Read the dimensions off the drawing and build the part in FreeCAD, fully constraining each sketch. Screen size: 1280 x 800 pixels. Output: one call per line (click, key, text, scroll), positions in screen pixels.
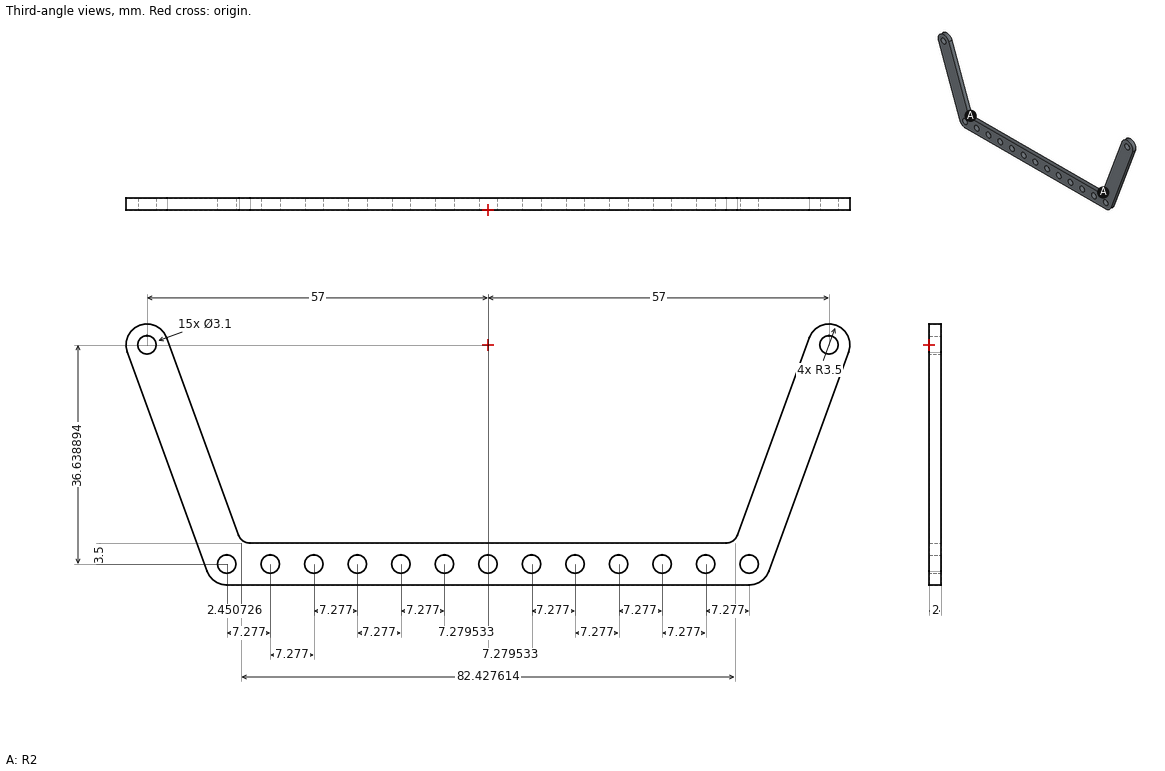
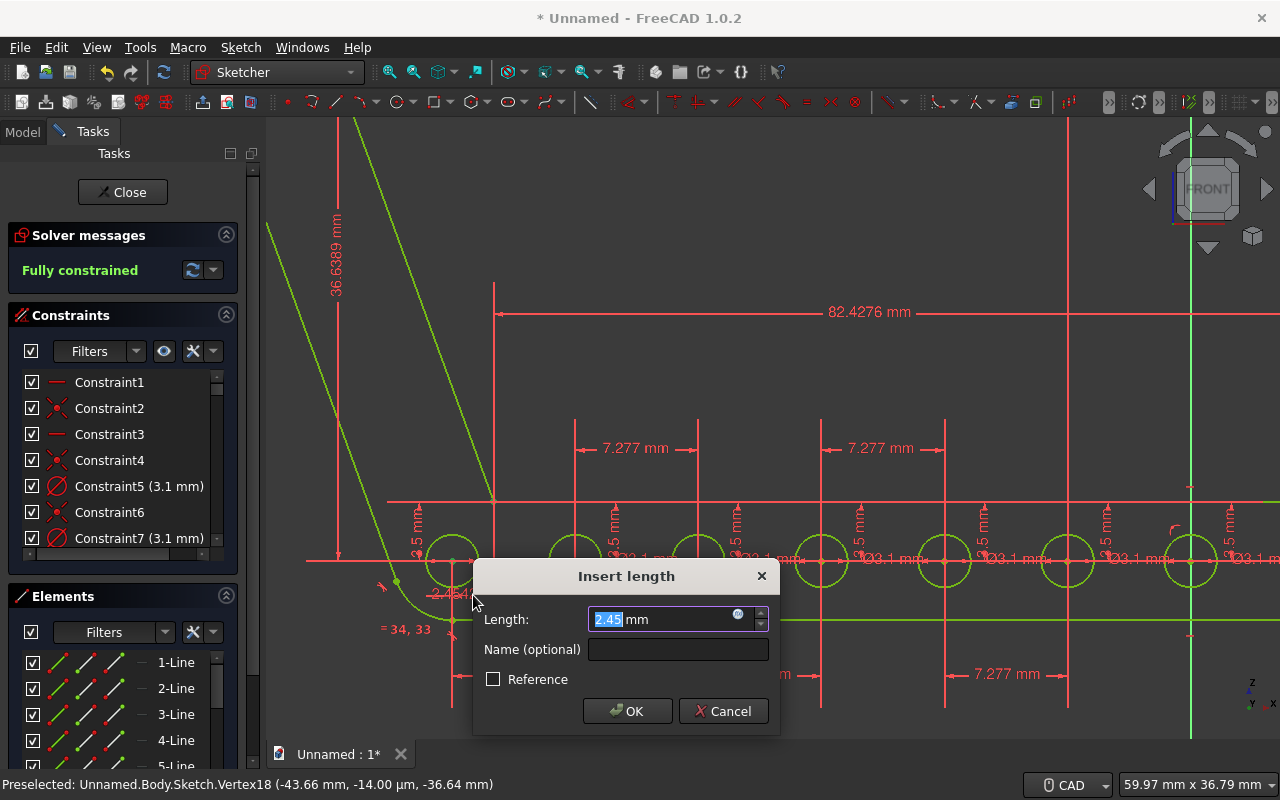
text(2.450726)
key(Return)
key(Escape)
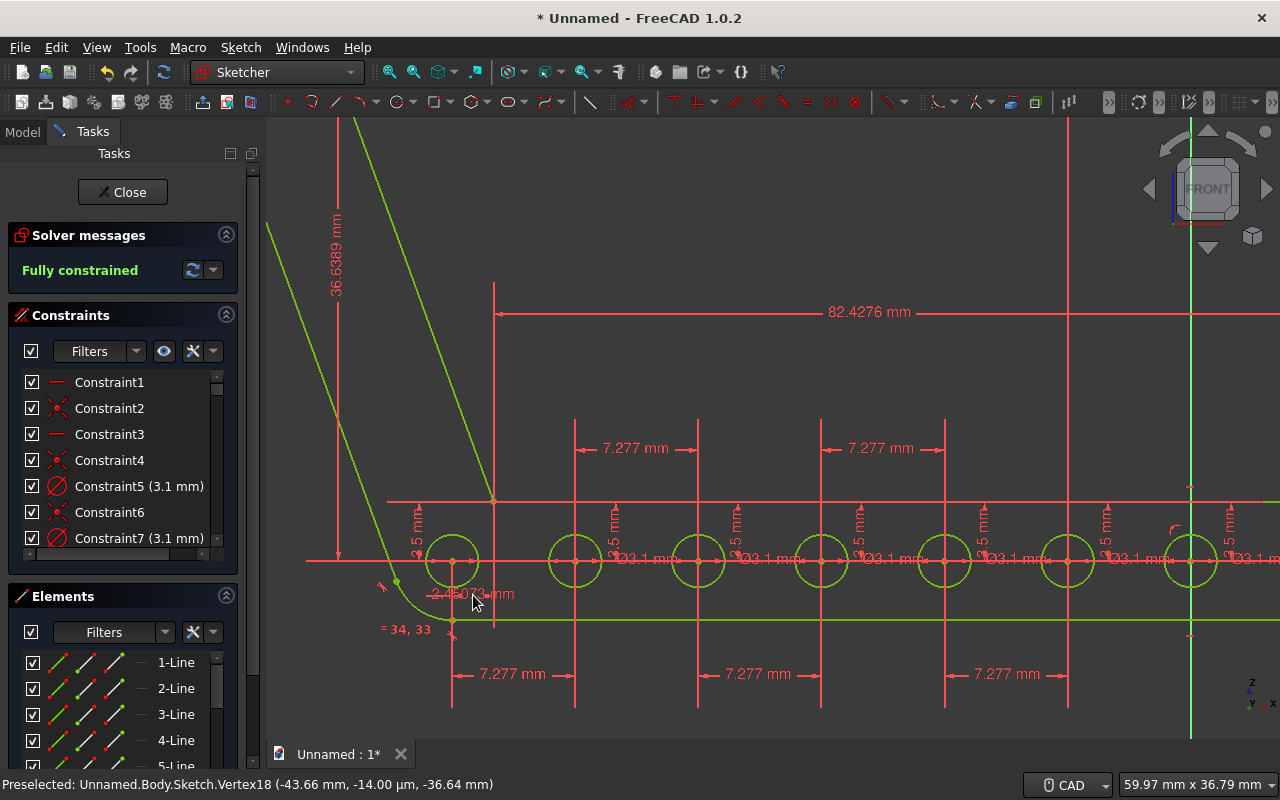
click(123, 192)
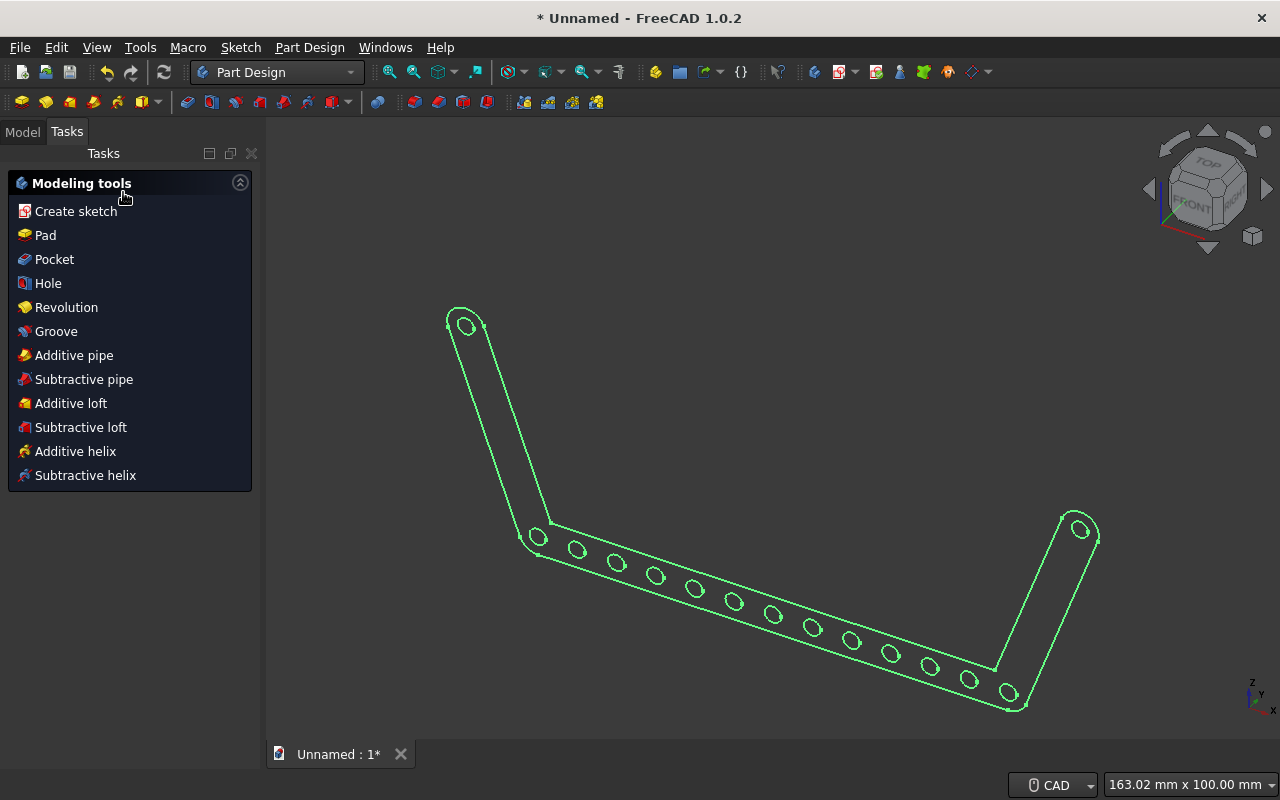
click(22, 102)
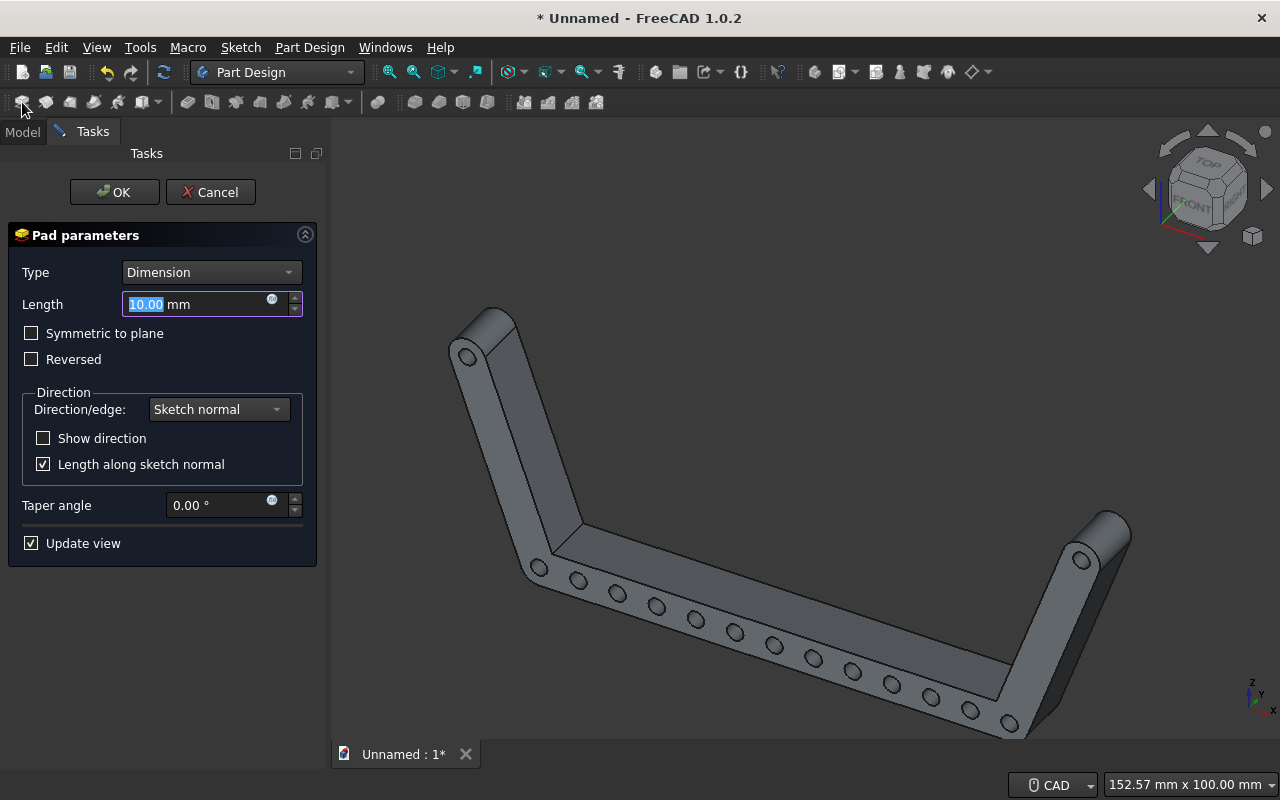
text(2)
key(Tab)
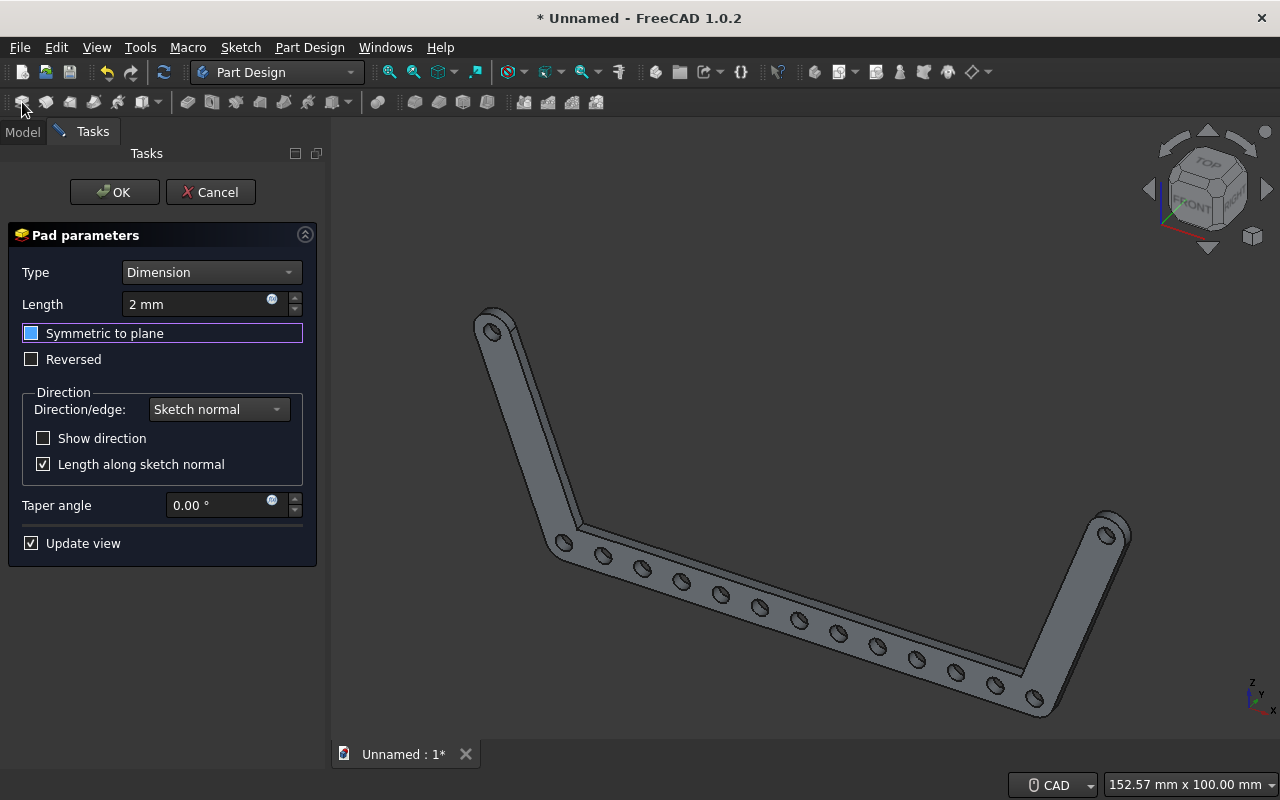
click(30, 359)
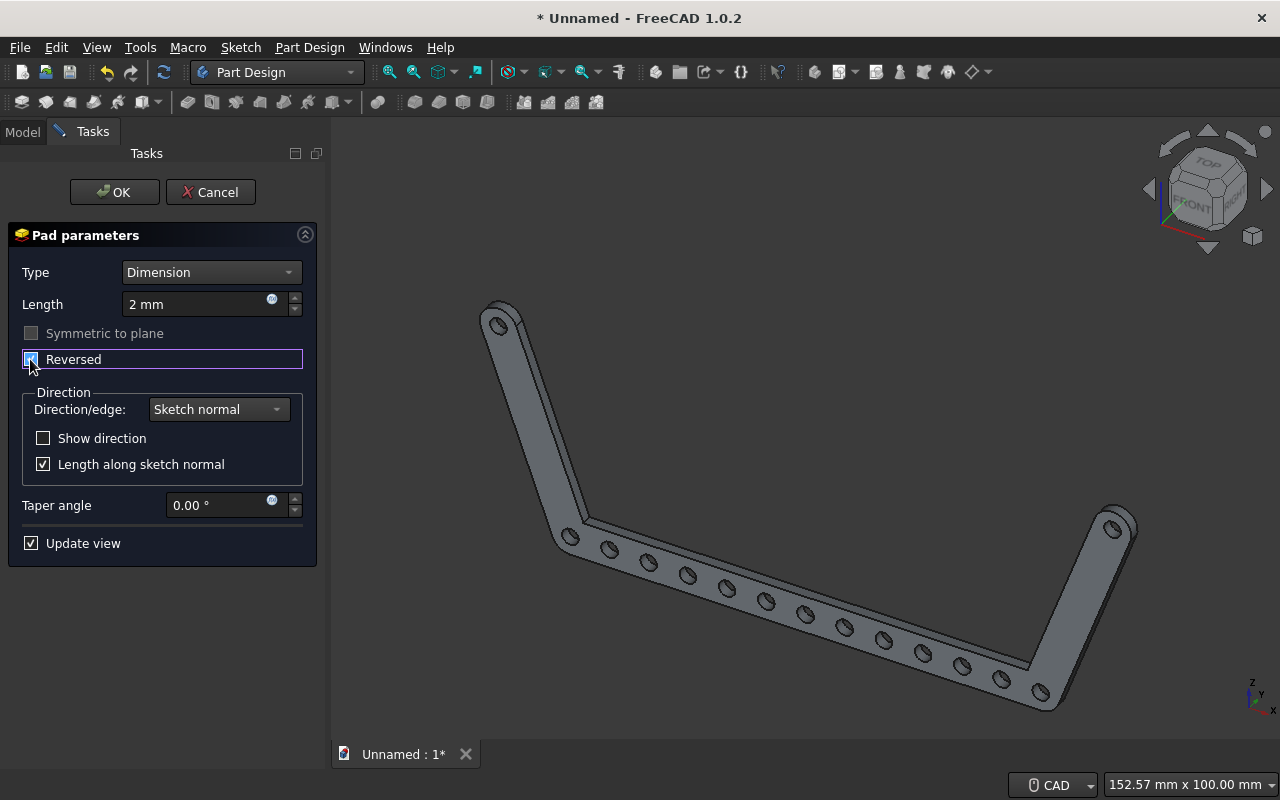
click(115, 192)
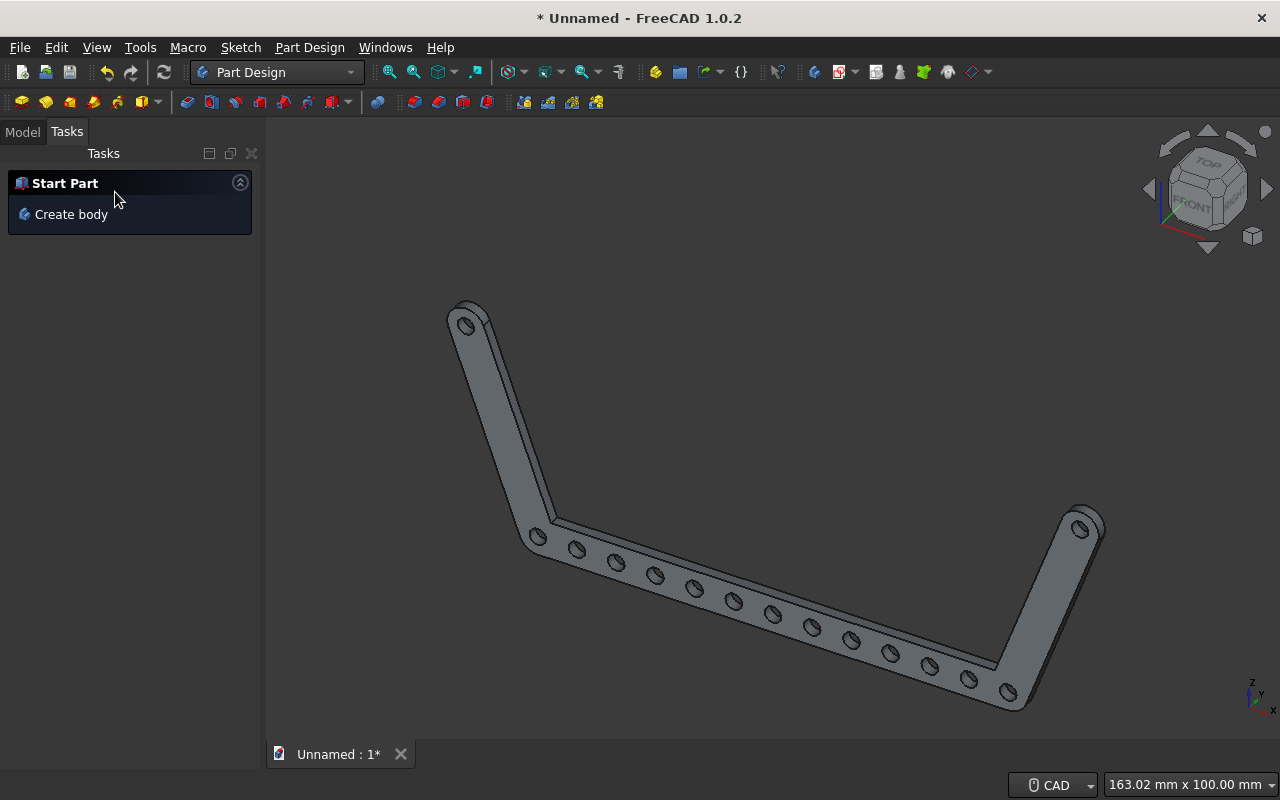
scroll(554, 519, up, 6)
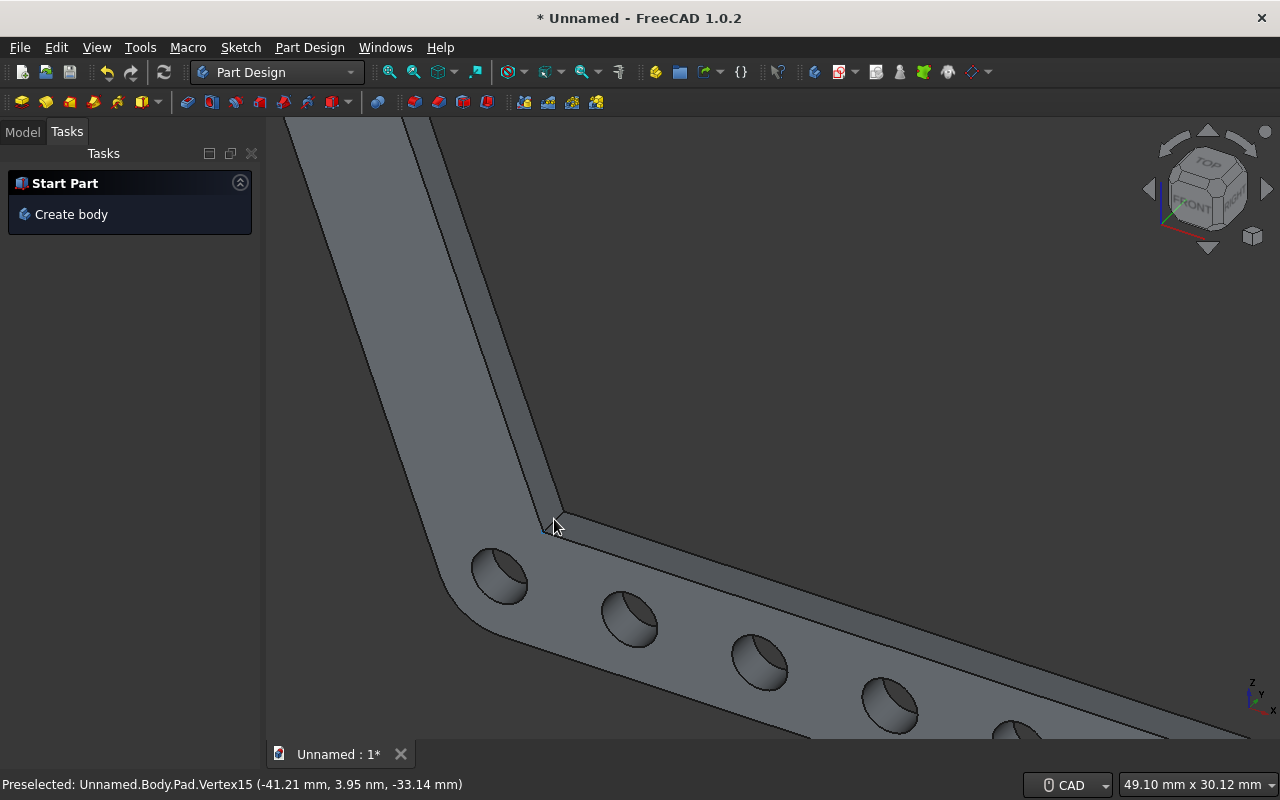
key(v)
key(f)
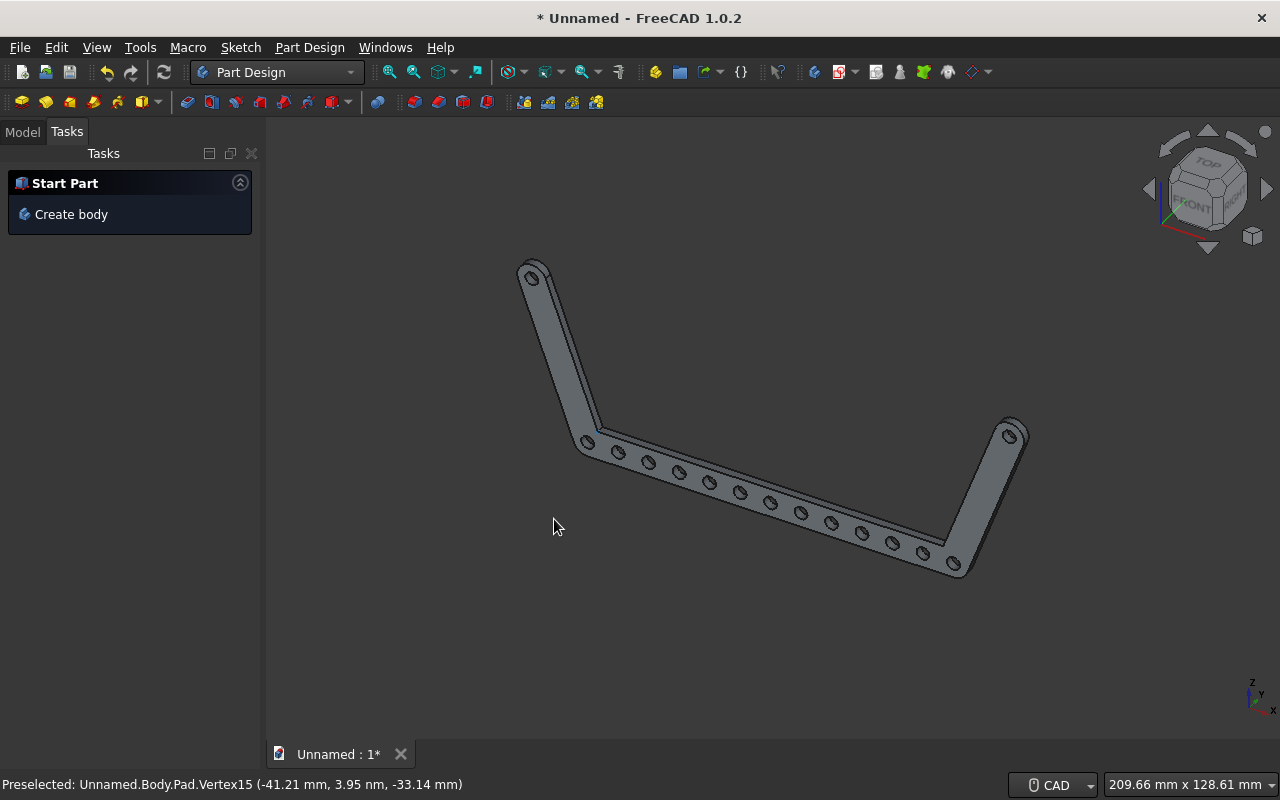
key(0)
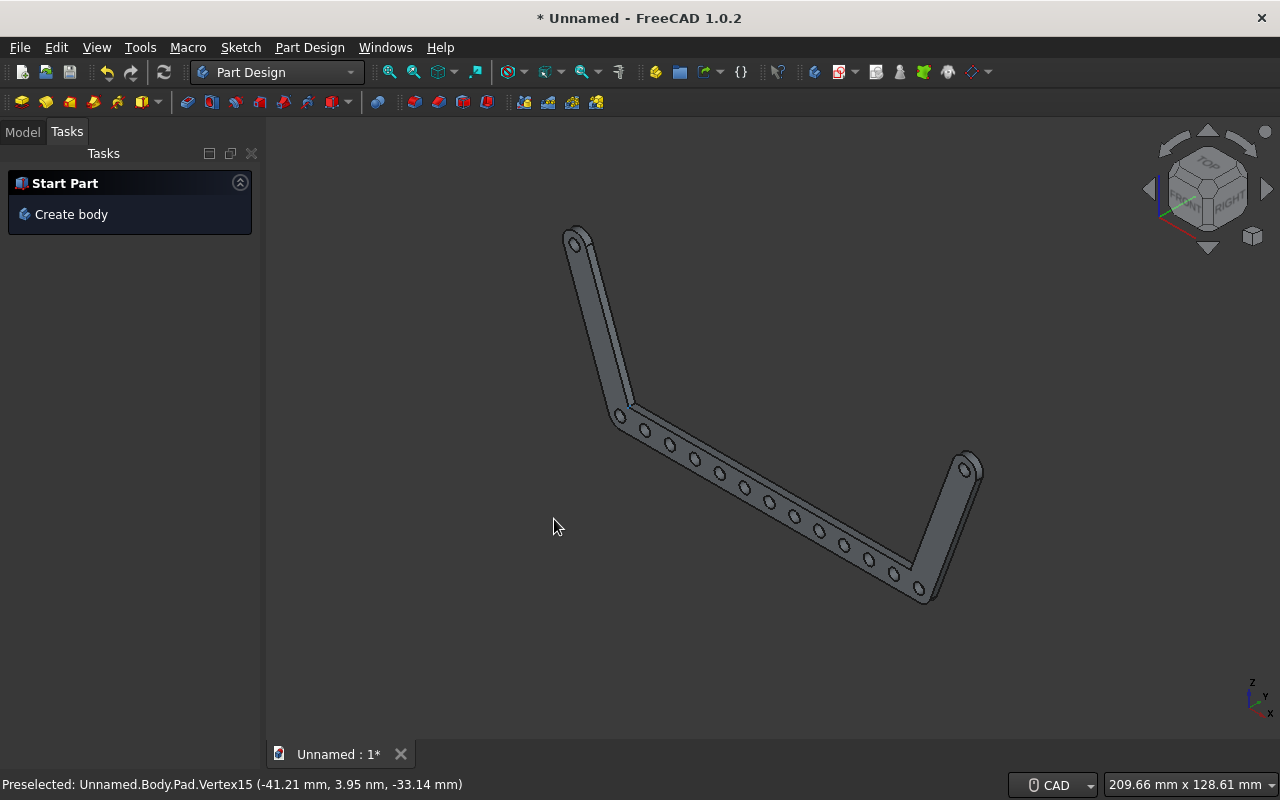
scroll(632, 404, up, 8)